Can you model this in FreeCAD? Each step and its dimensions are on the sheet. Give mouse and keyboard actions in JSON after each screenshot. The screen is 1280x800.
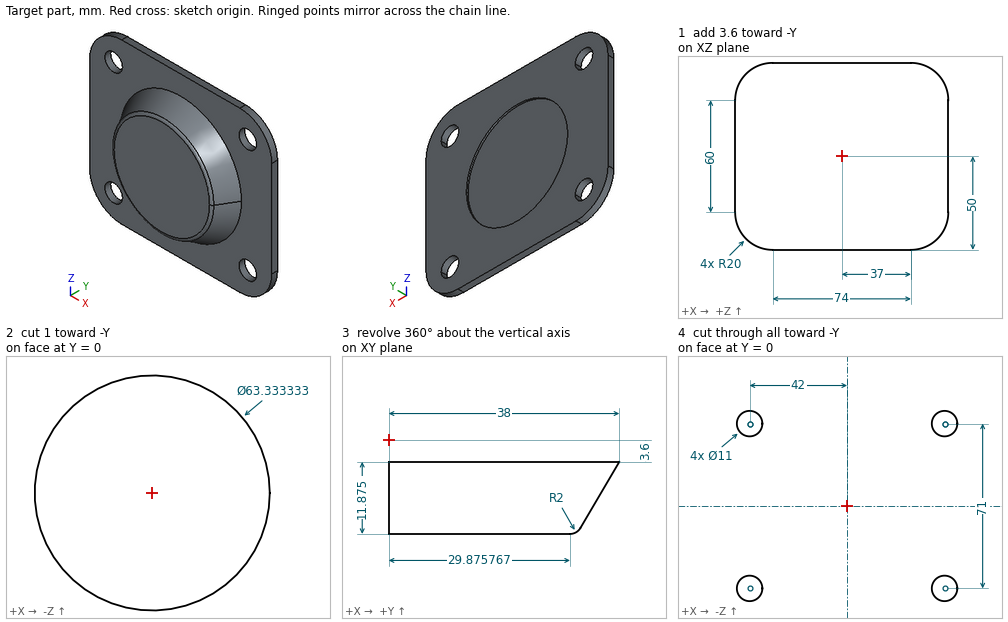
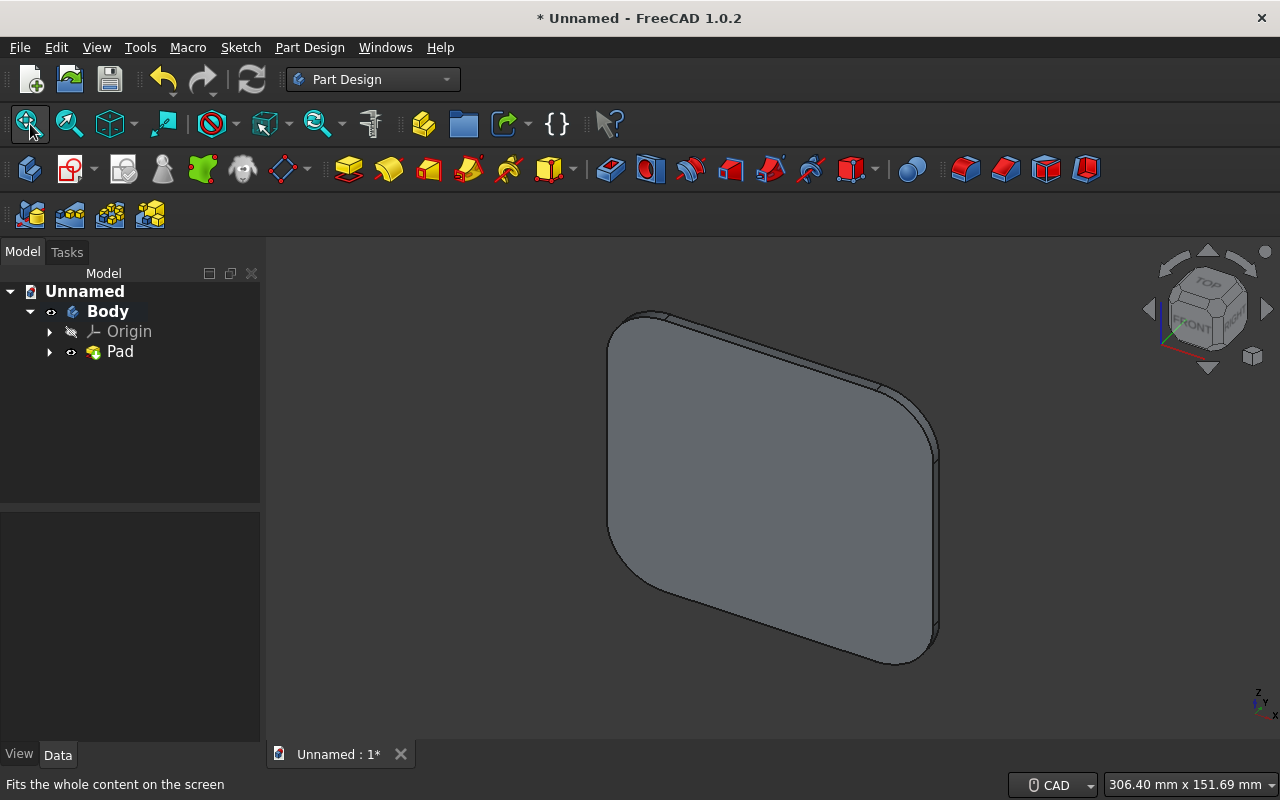
{"action": "key", "text": "4"}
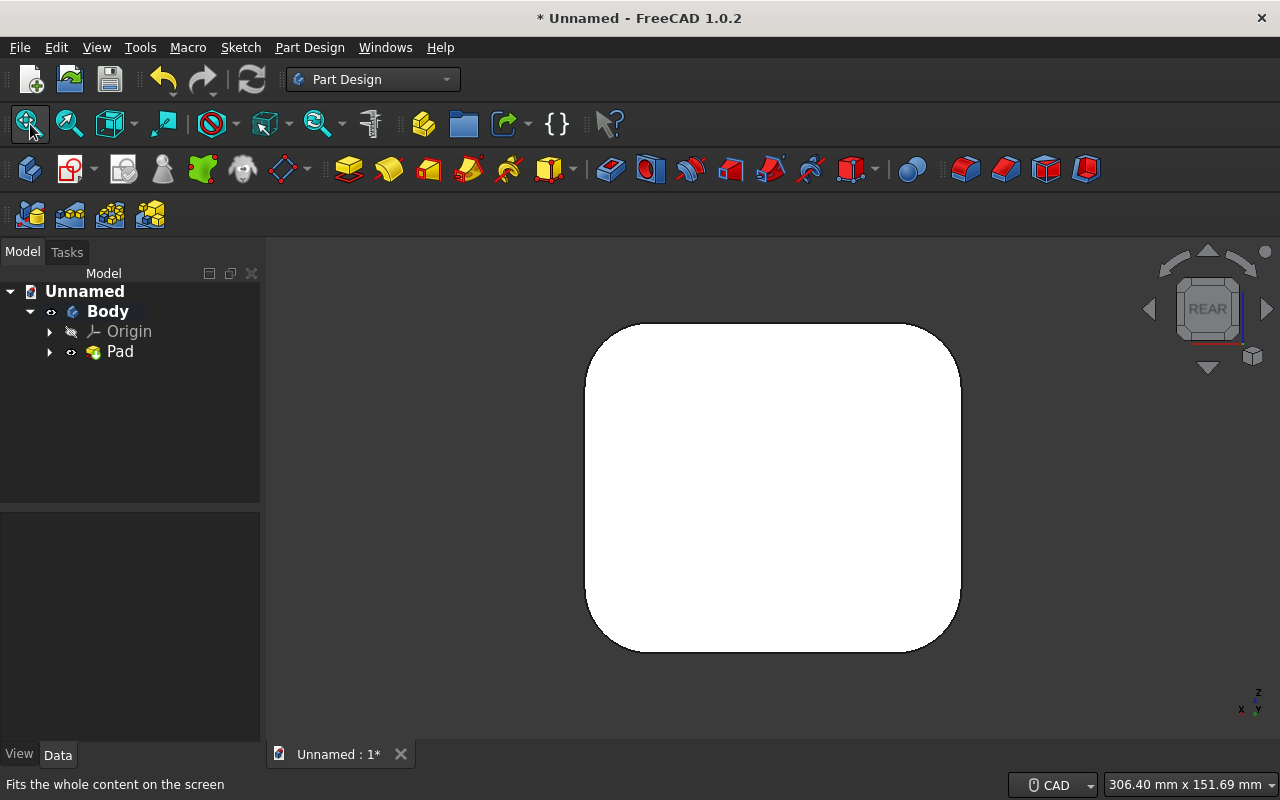
{"action": "left_click", "coordinate": [773, 487]}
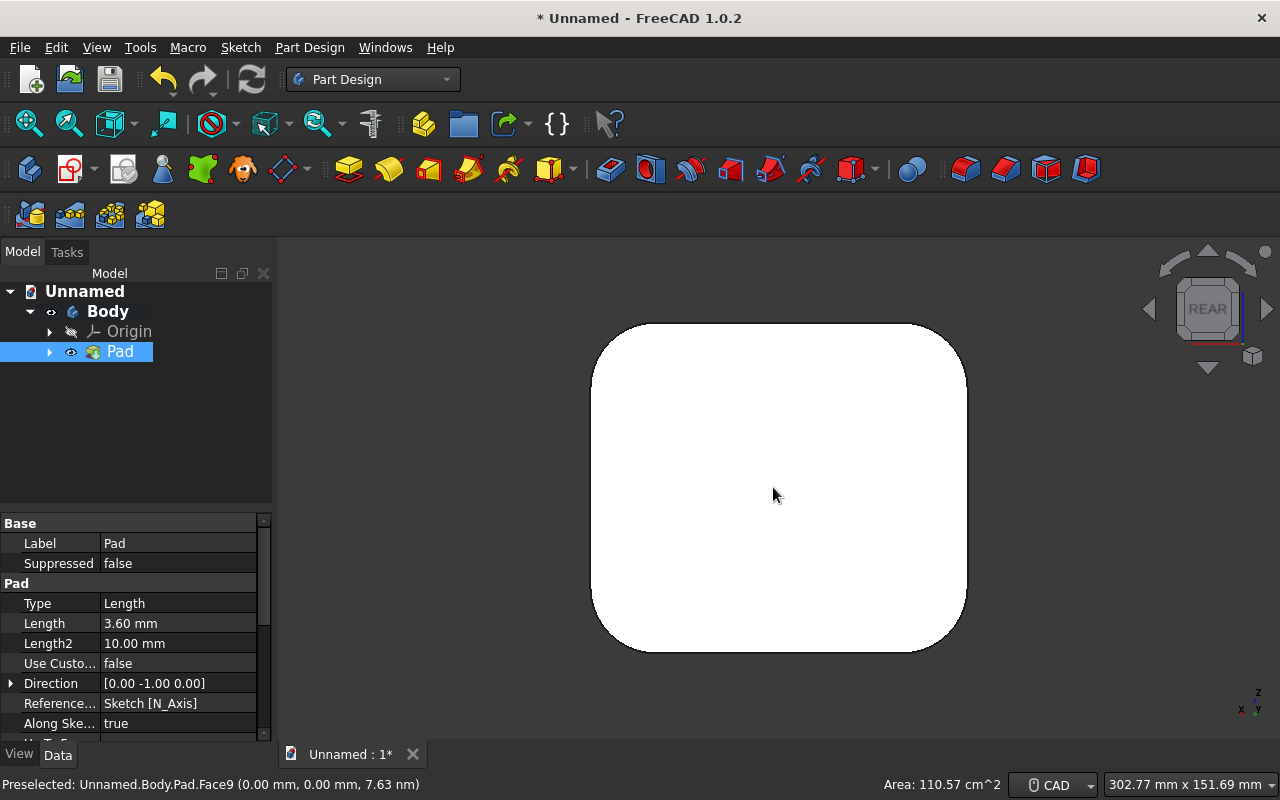
{"action": "left_click", "coordinate": [70, 170]}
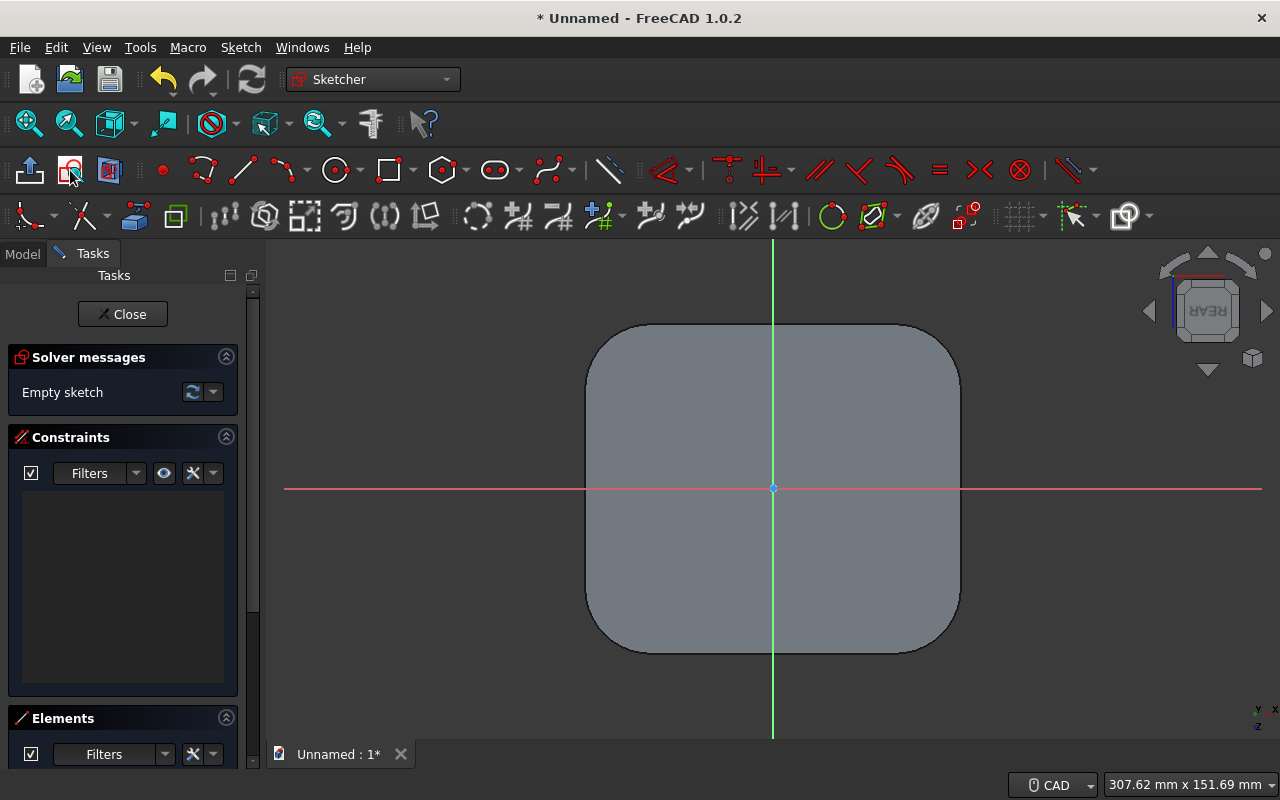
{"action": "scroll", "coordinate": [912, 489], "scroll_direction": "up", "scroll_amount": 2}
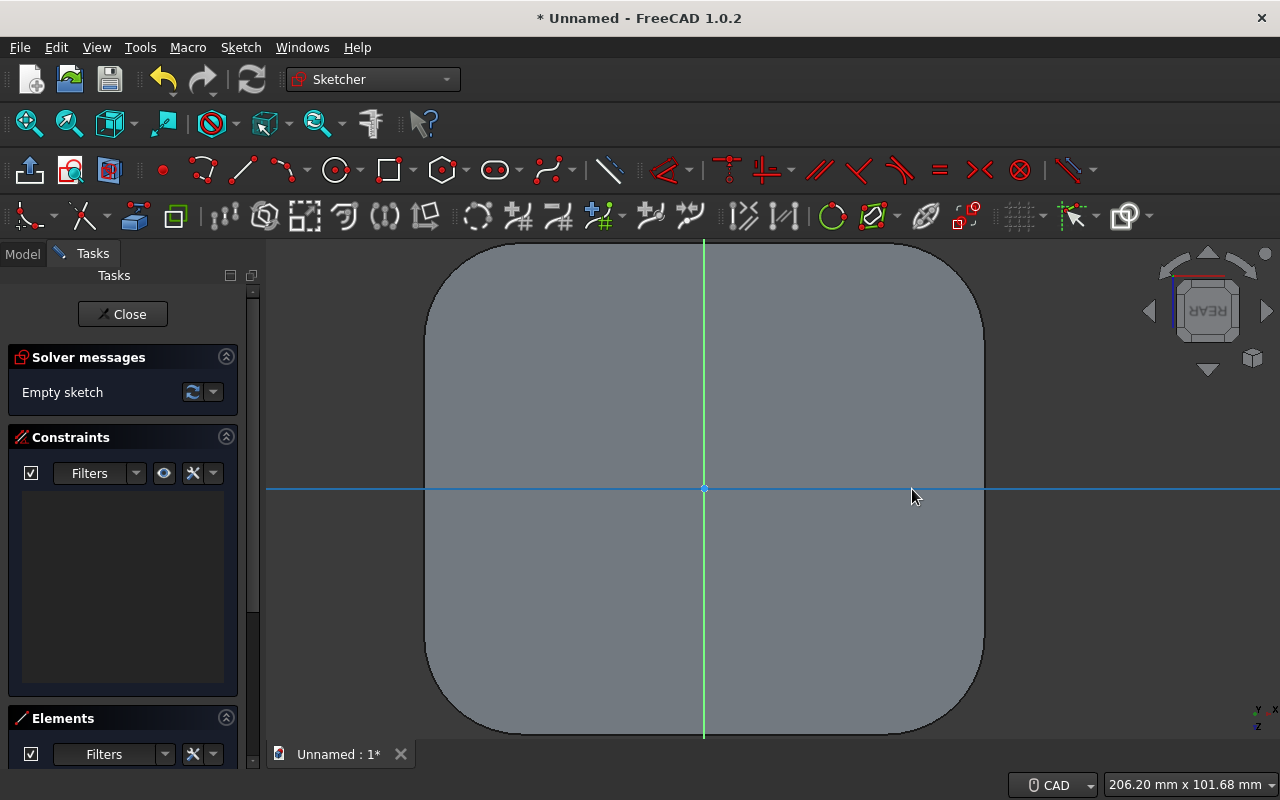
{"action": "left_click", "coordinate": [336, 170]}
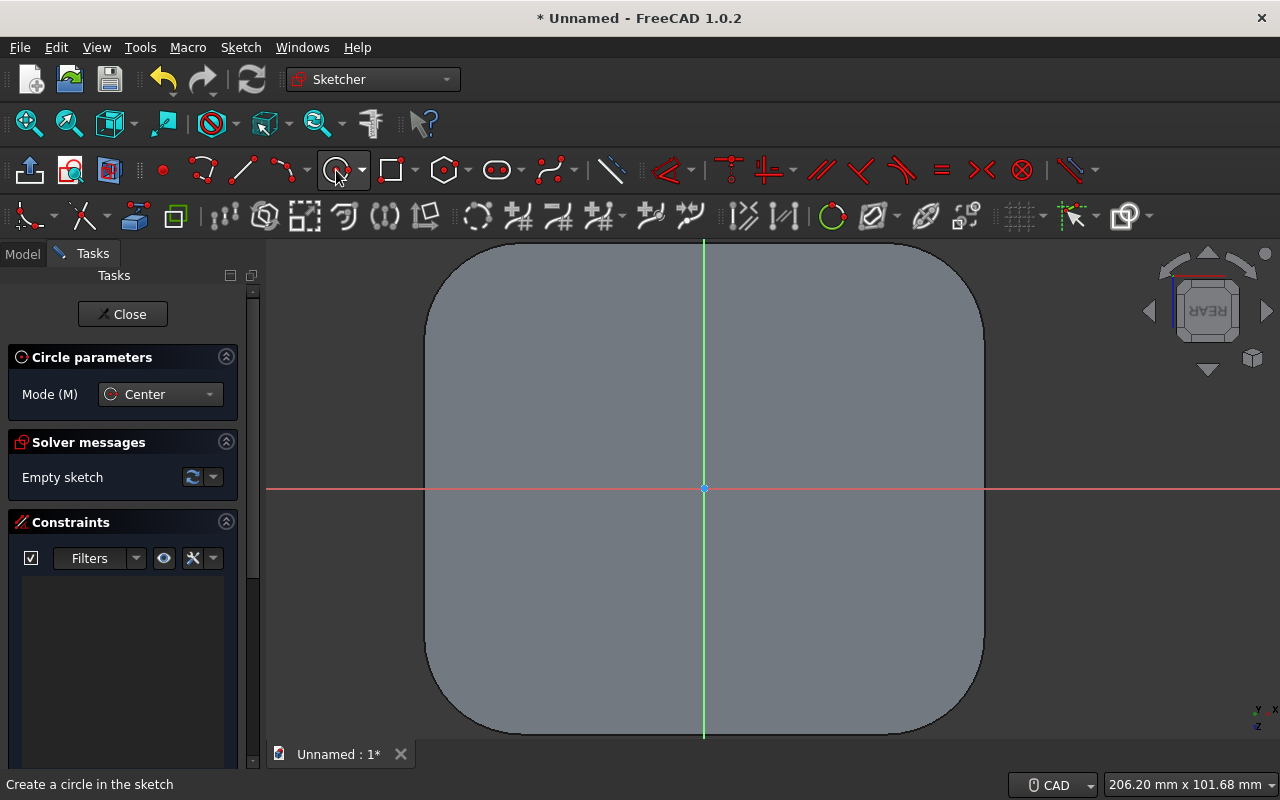
{"action": "left_click", "coordinate": [704, 489]}
{"action": "mouse_move", "coordinate": [814, 379]}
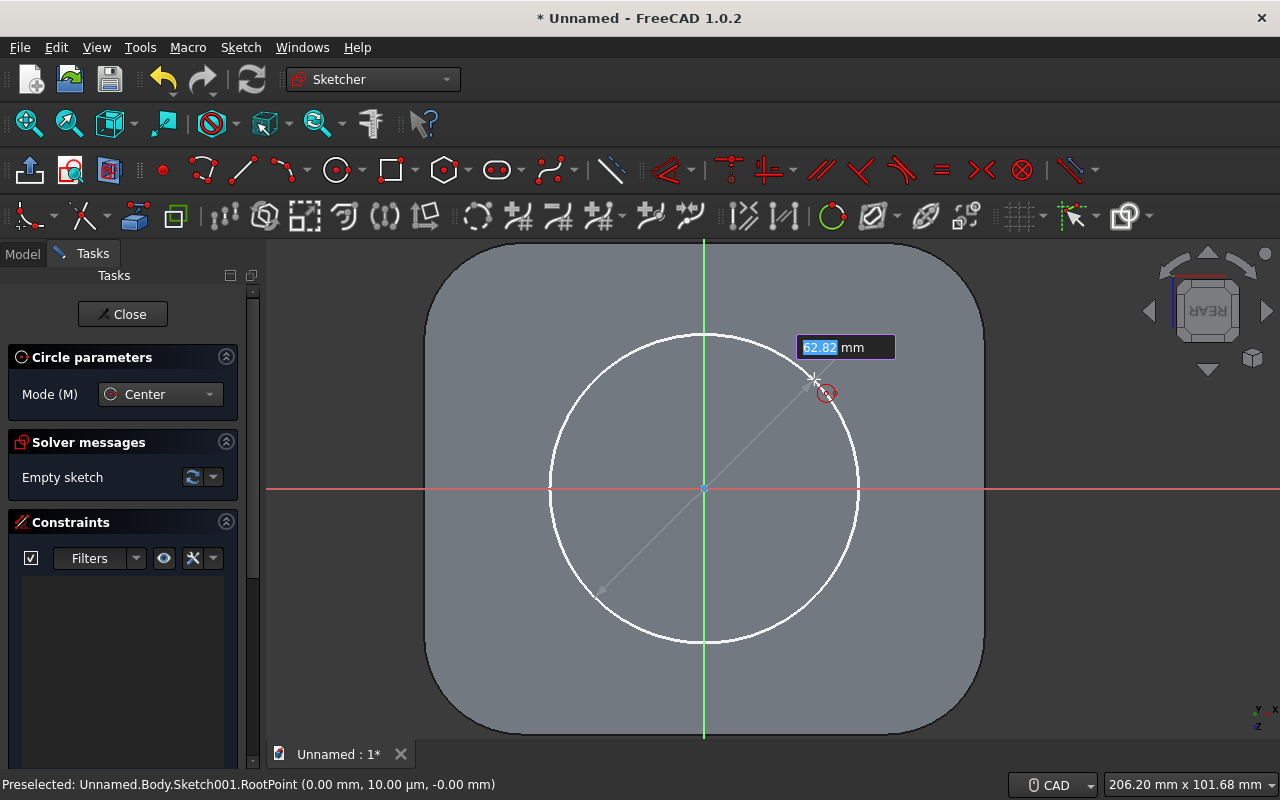
{"action": "type", "text": "63.333333"}
{"action": "key", "text": "Return"}
{"action": "key", "text": "Escape"}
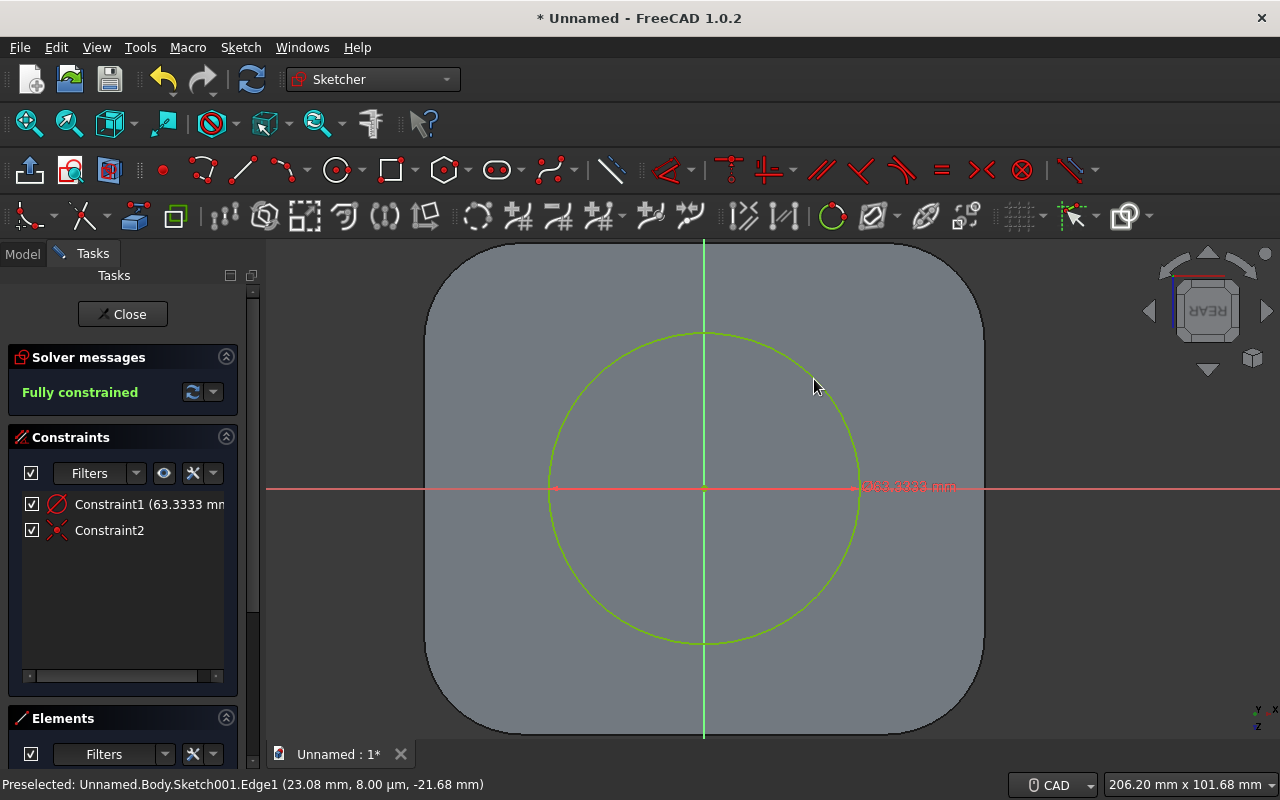
{"action": "left_click", "coordinate": [123, 314]}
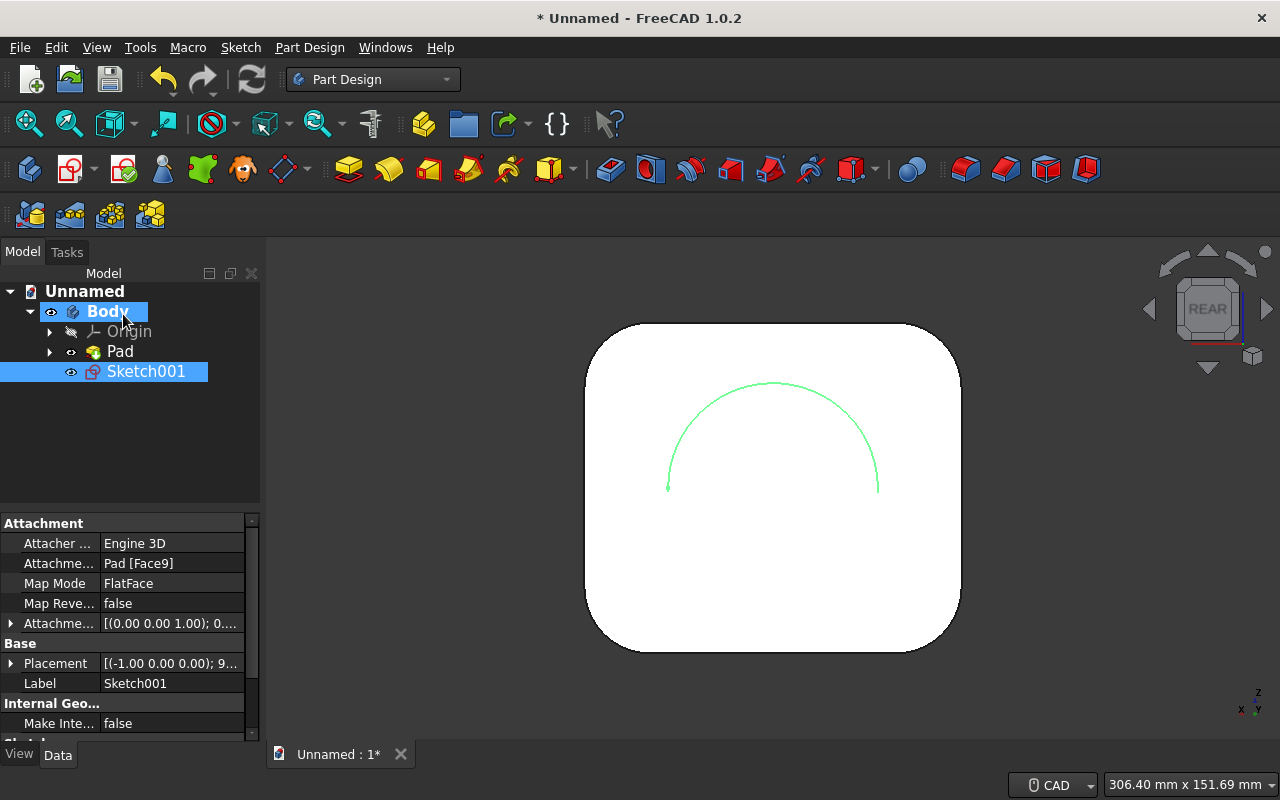
{"action": "left_click", "coordinate": [612, 170]}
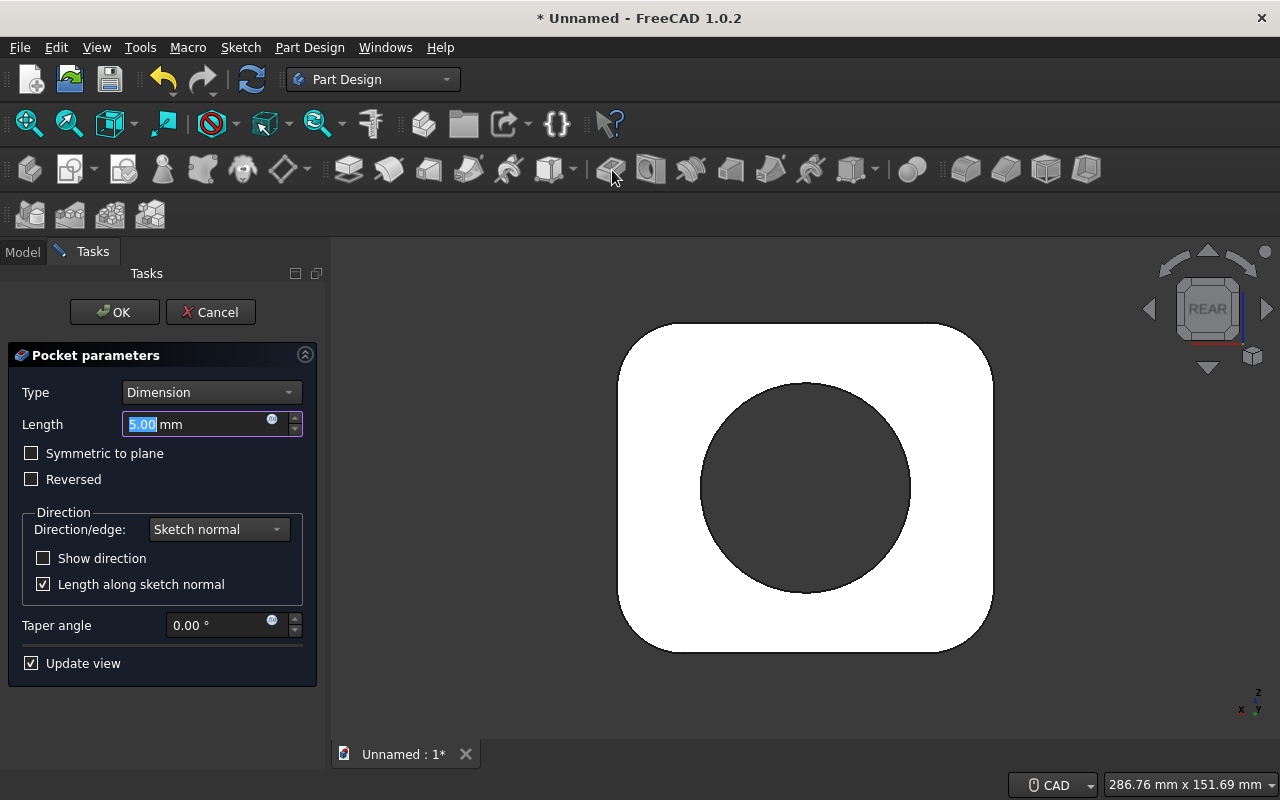
{"action": "type", "text": "1"}
{"action": "key", "text": "Tab"}